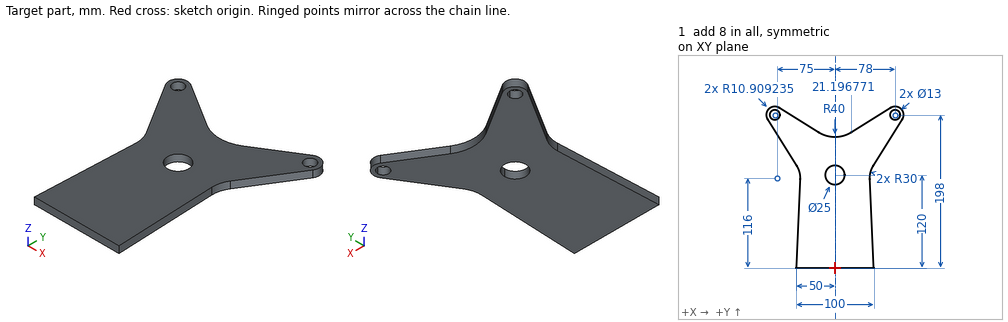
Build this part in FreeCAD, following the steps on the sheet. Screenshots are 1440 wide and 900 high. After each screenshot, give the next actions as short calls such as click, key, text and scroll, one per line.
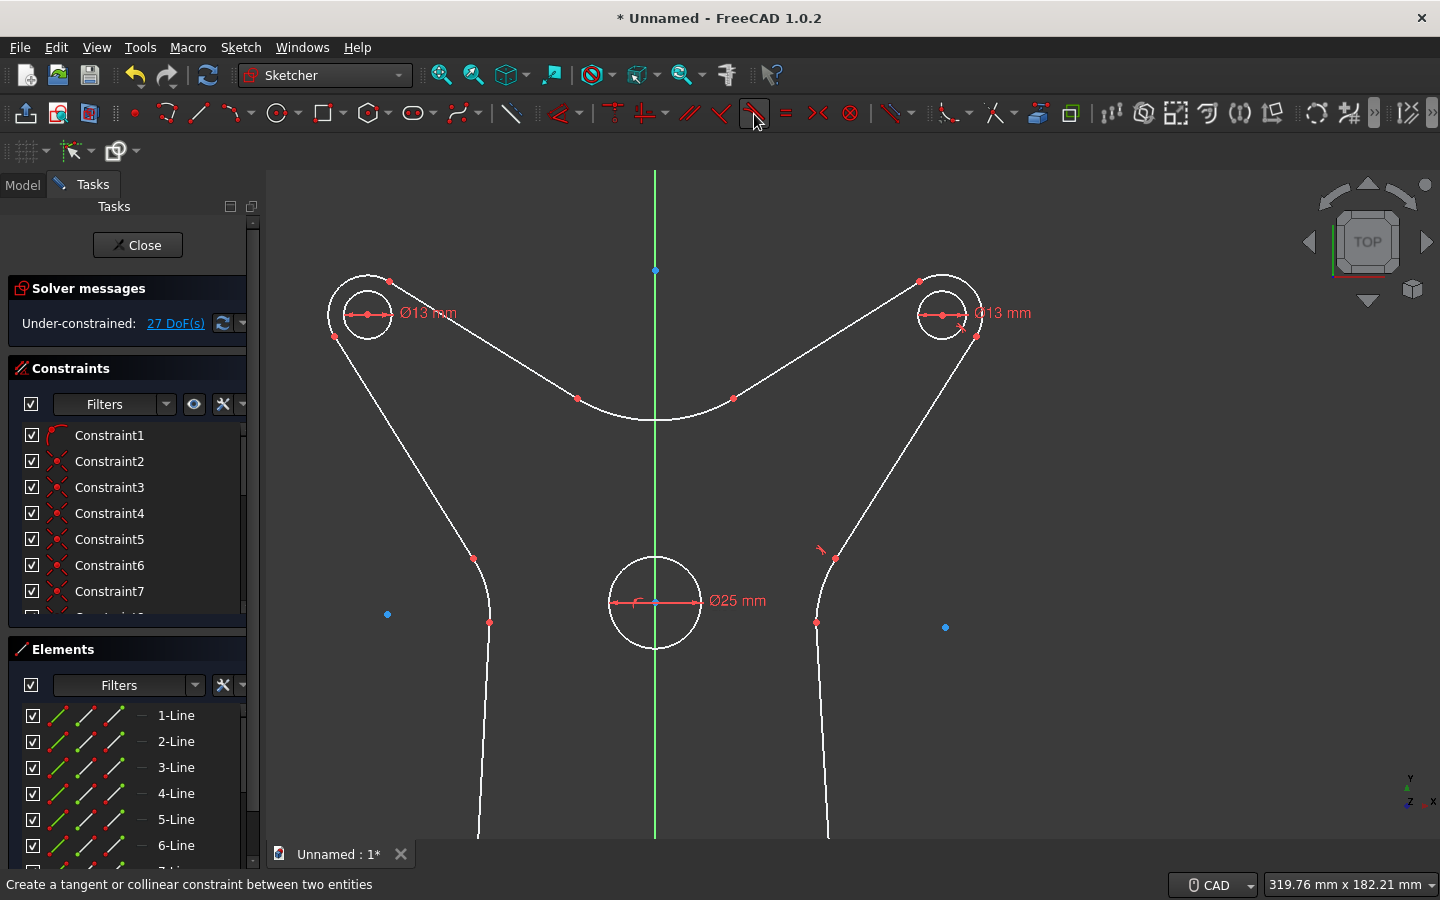
click(864, 317)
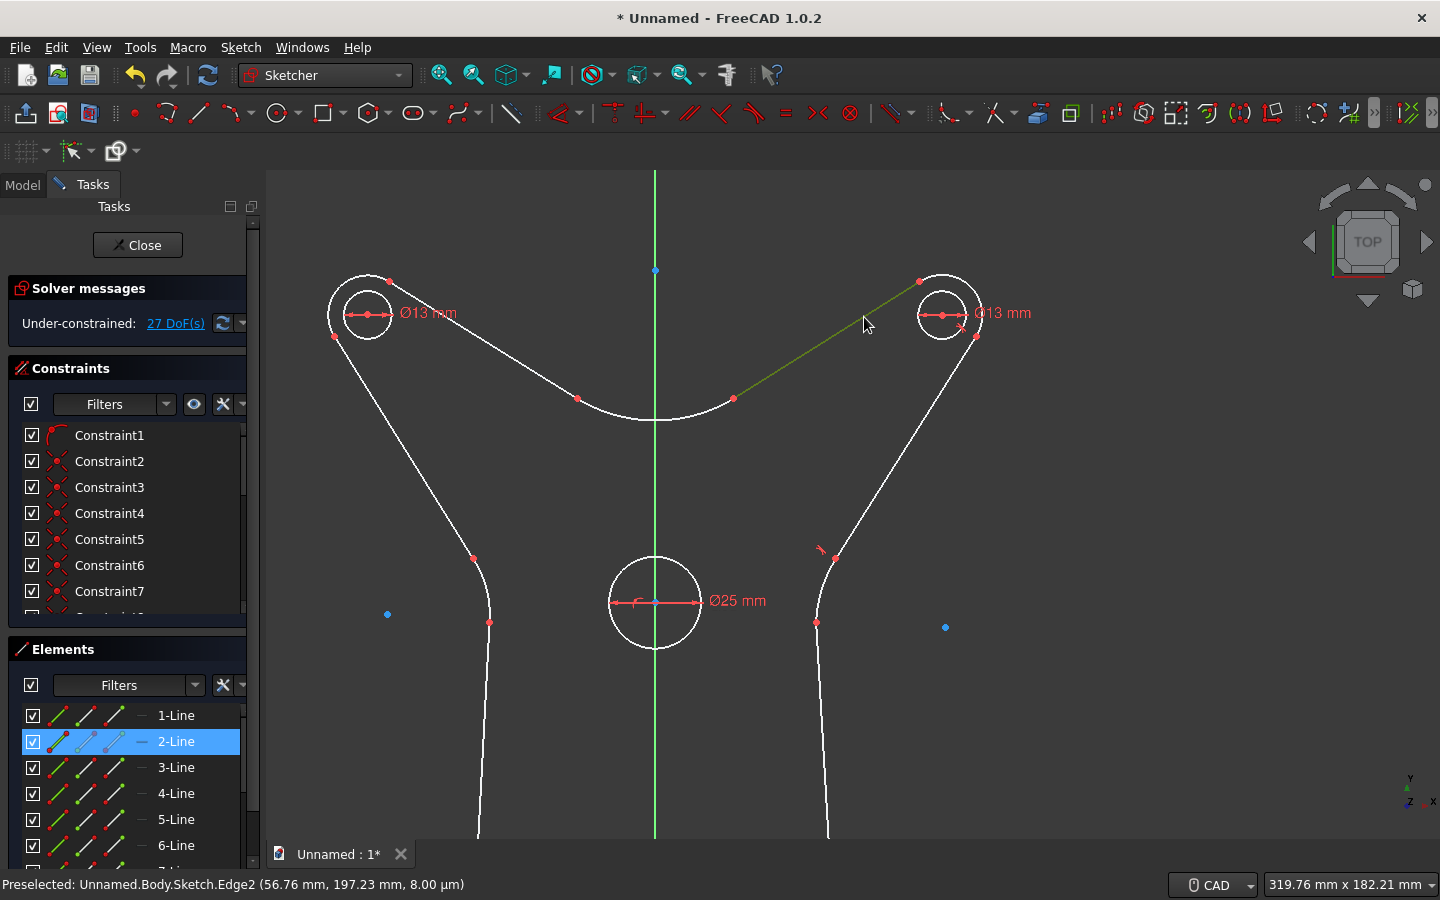
click(981, 305)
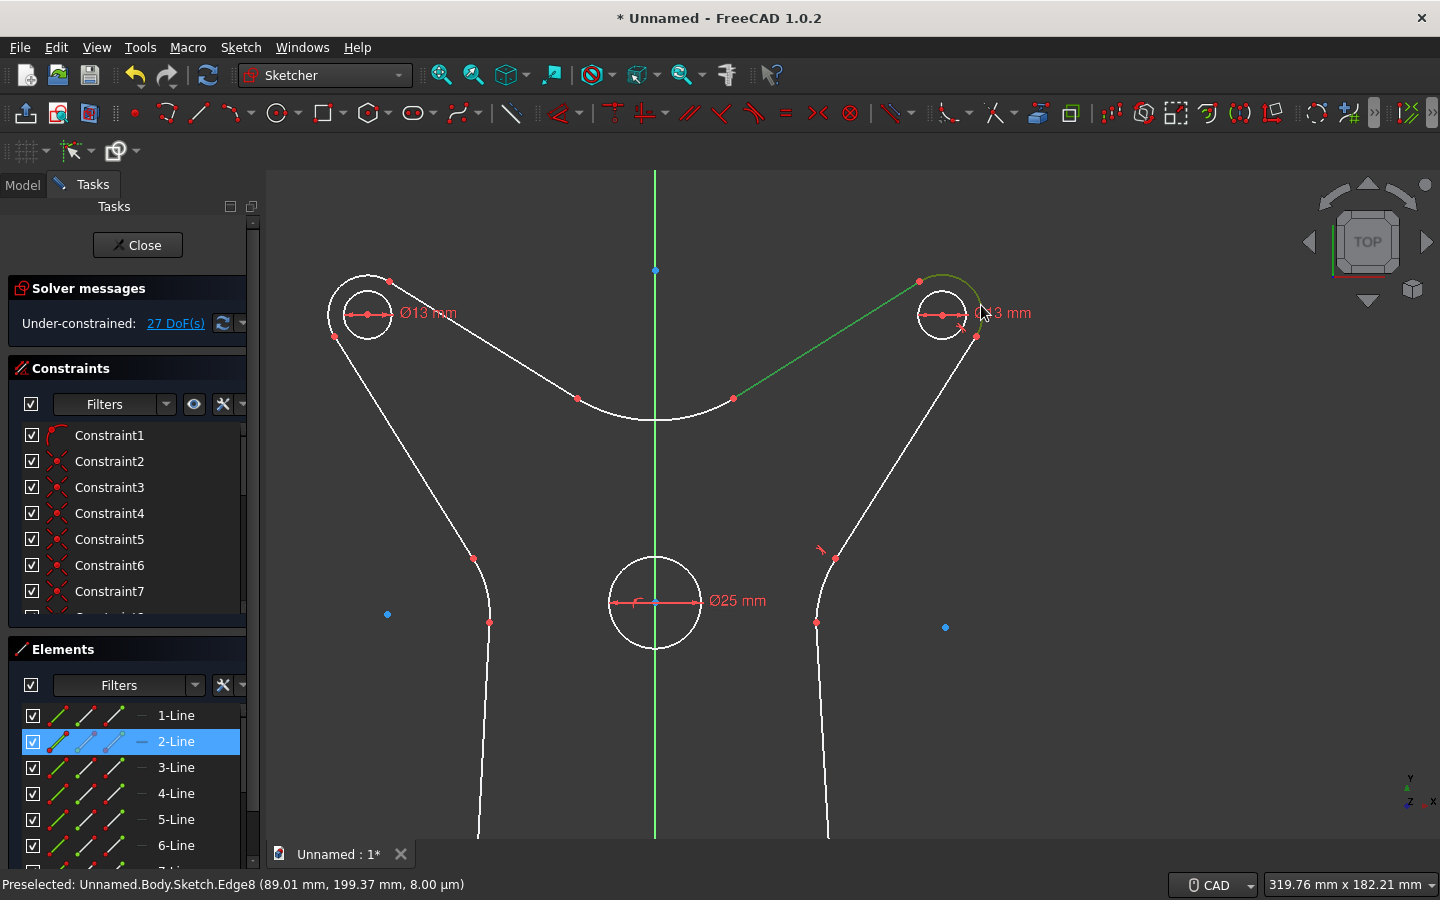
click(754, 114)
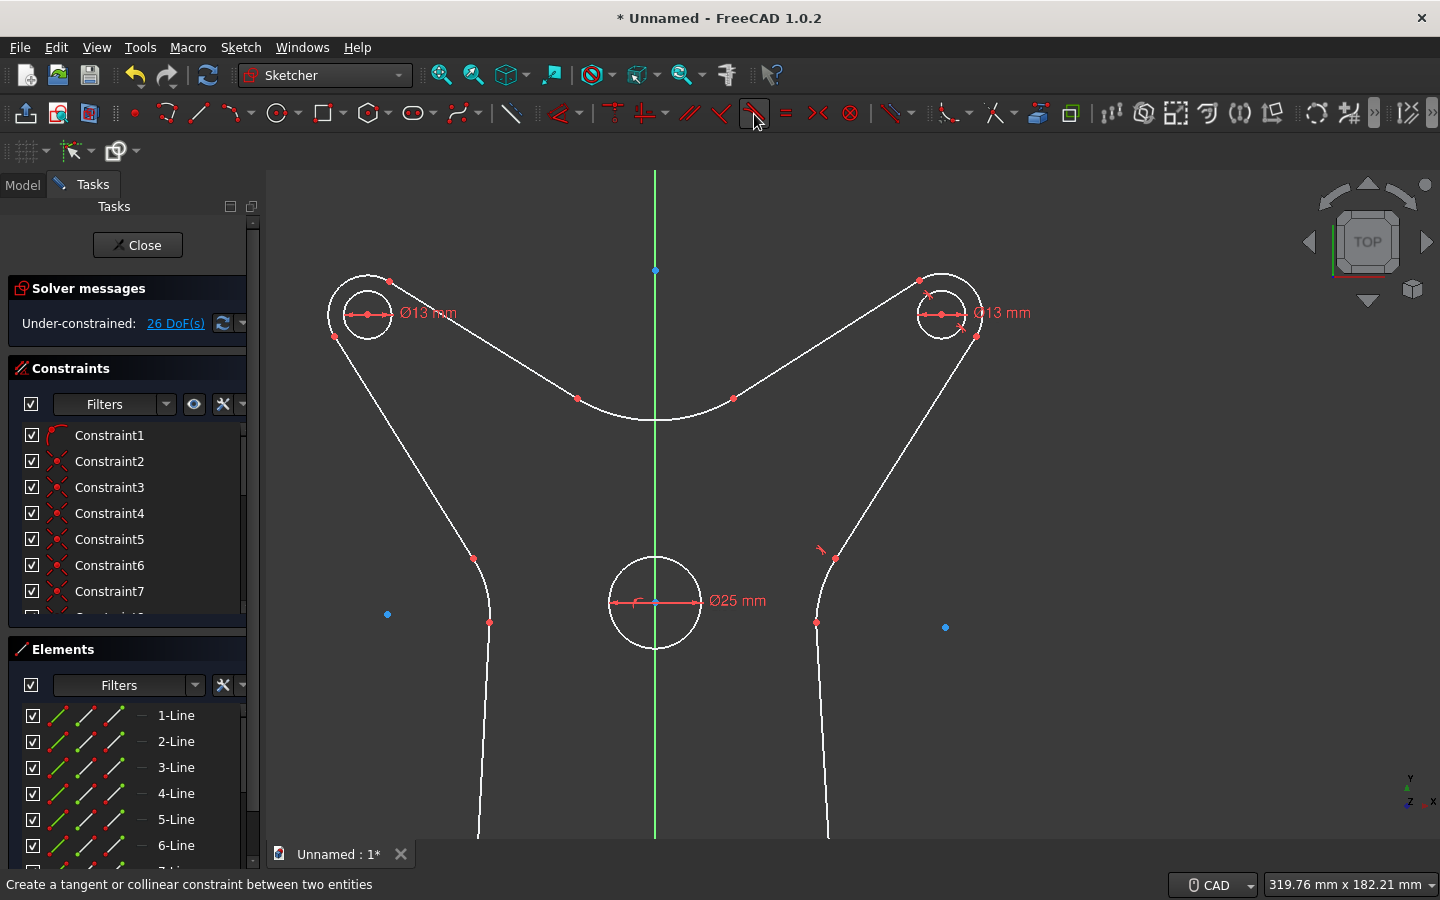
click(864, 316)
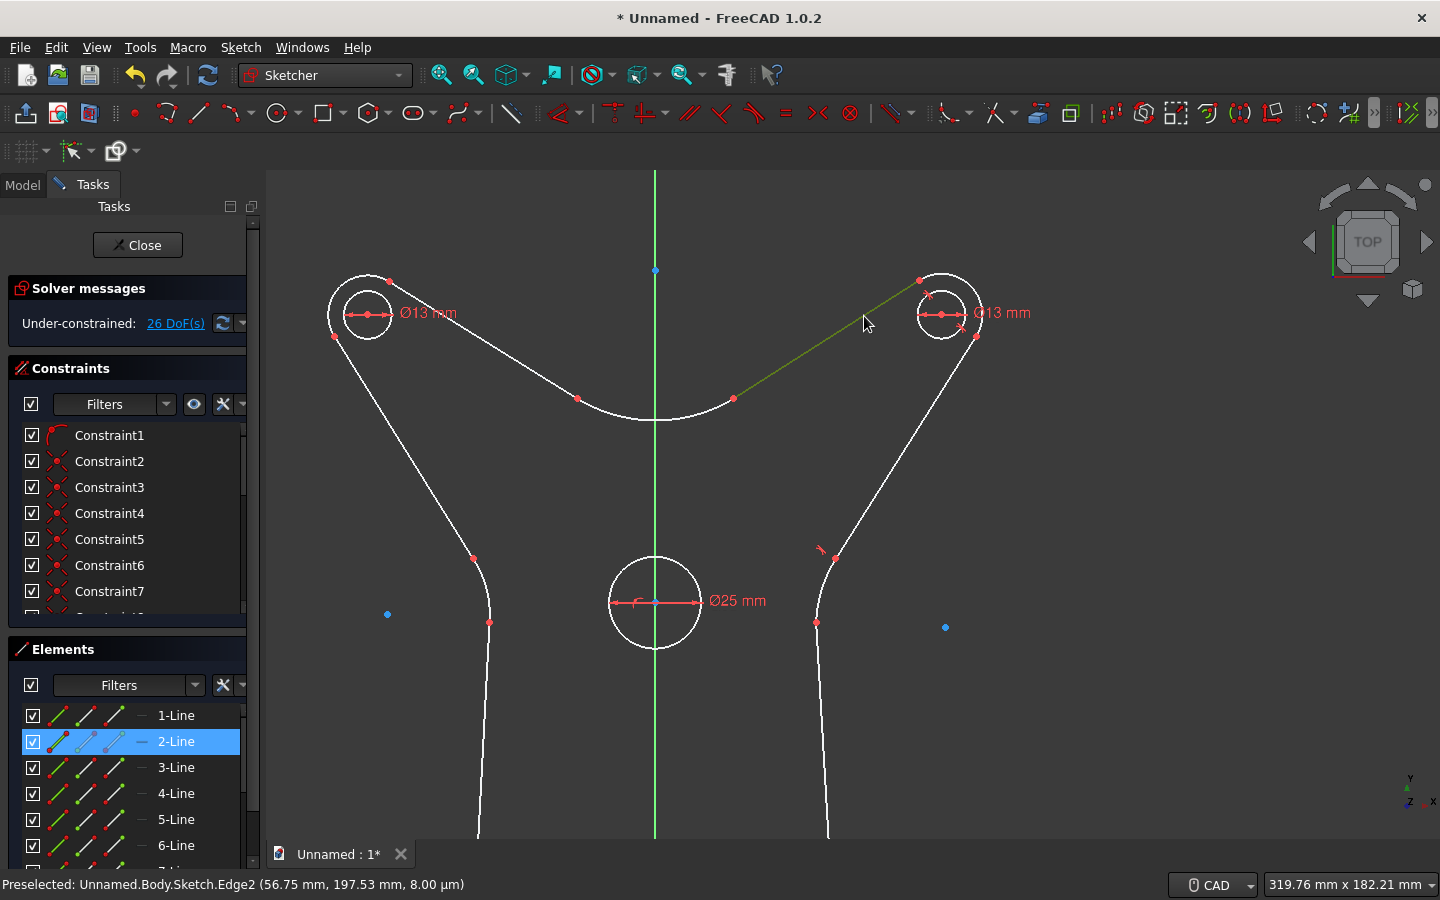
click(623, 417)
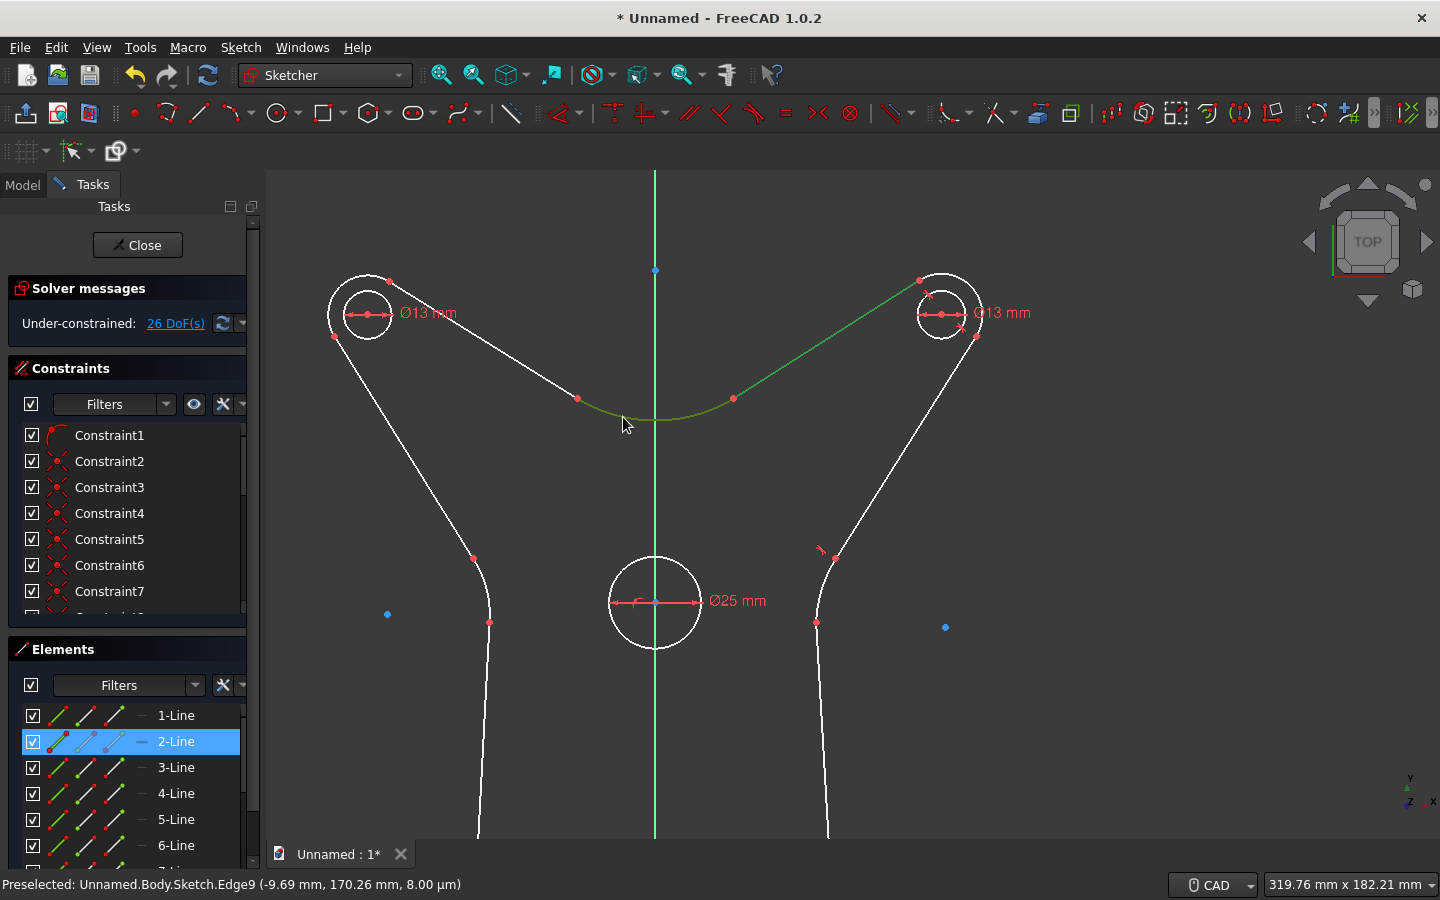
click(754, 114)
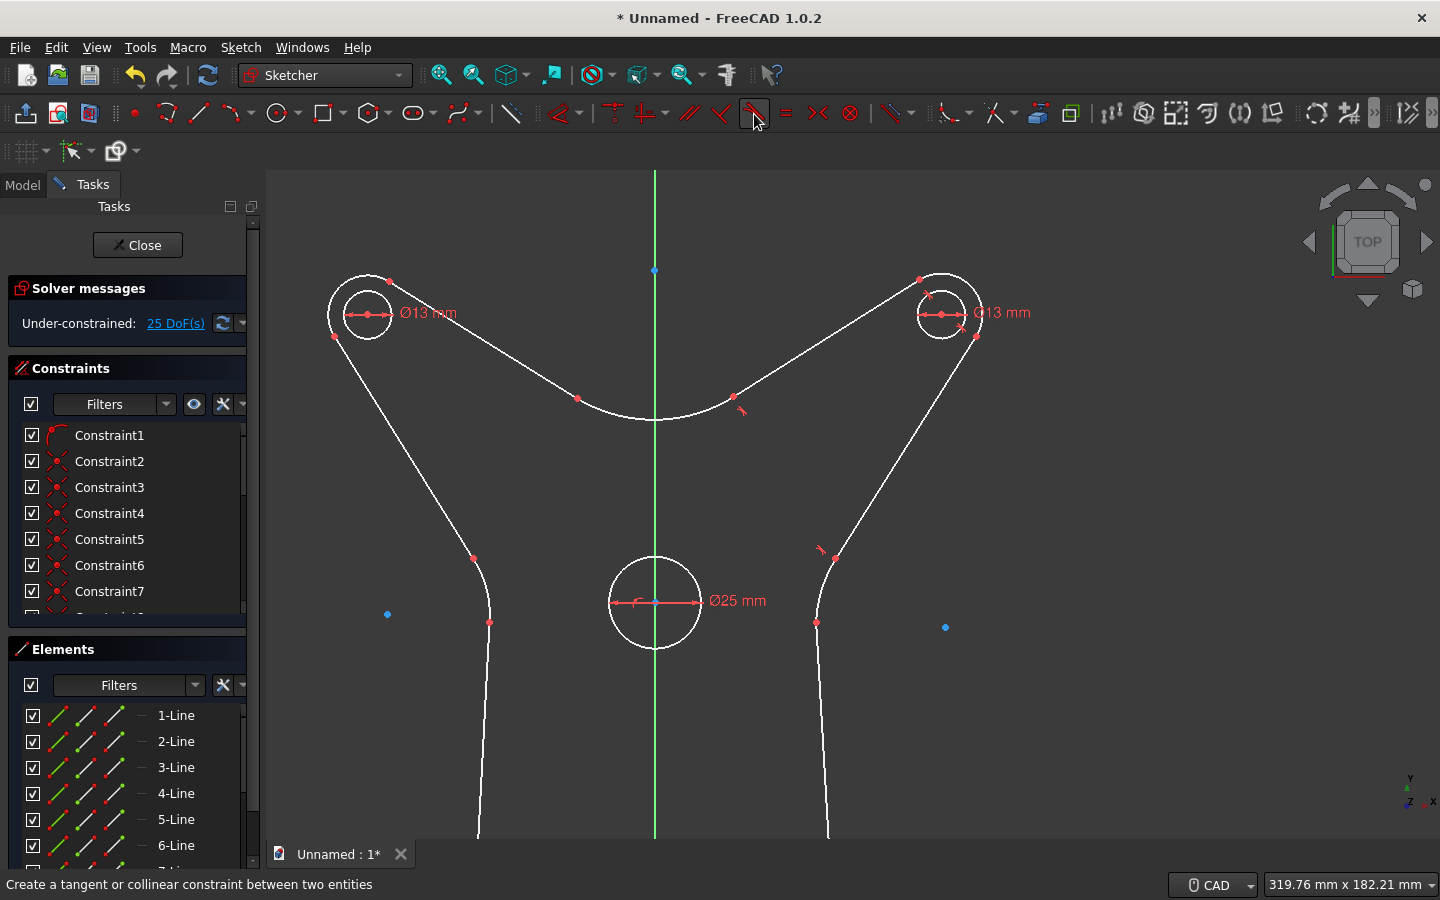
click(521, 363)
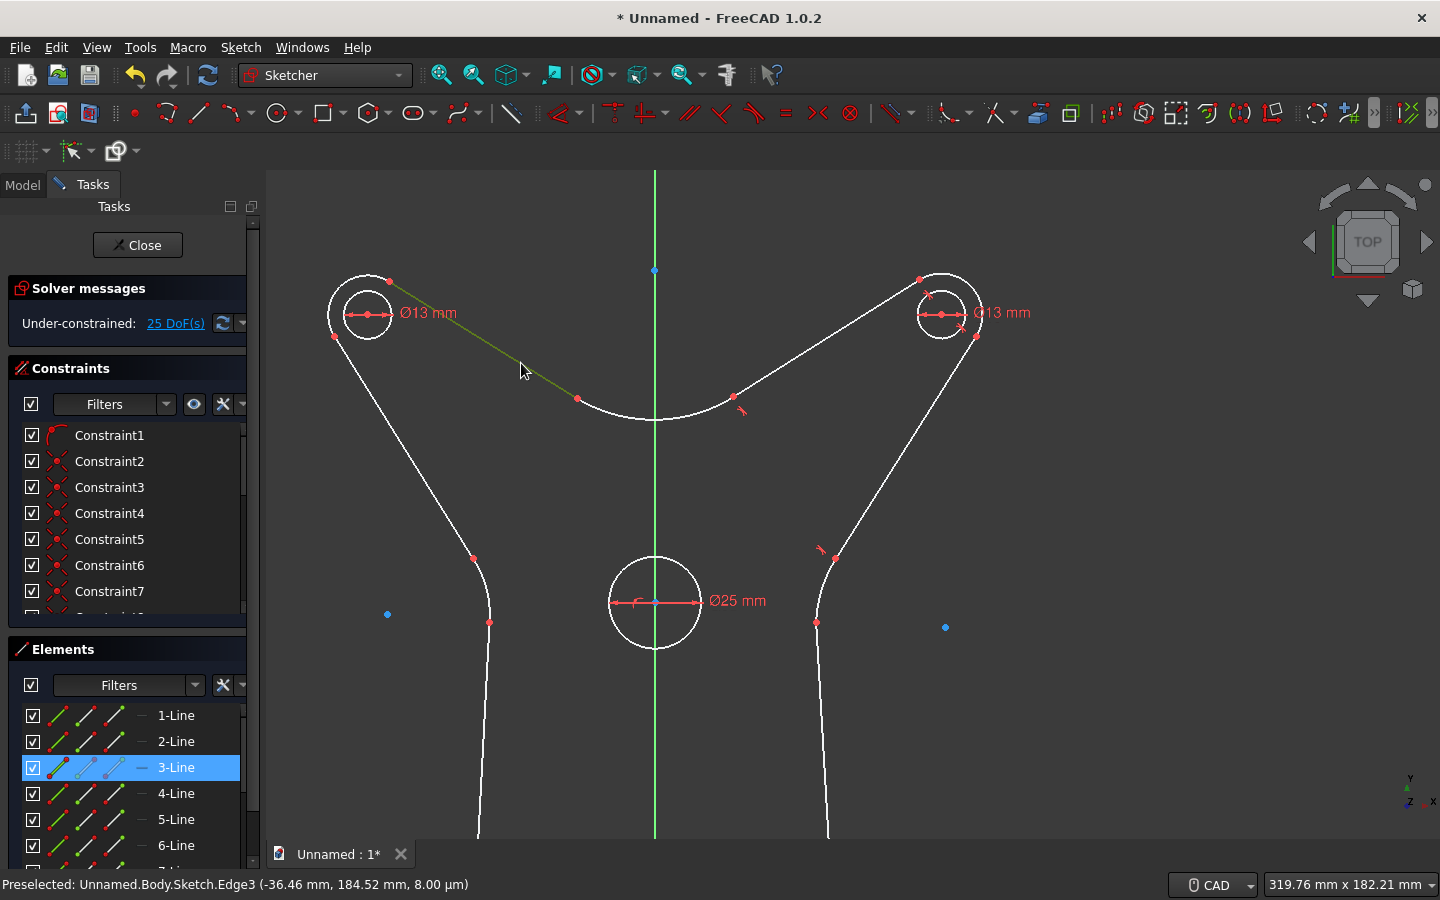
click(623, 417)